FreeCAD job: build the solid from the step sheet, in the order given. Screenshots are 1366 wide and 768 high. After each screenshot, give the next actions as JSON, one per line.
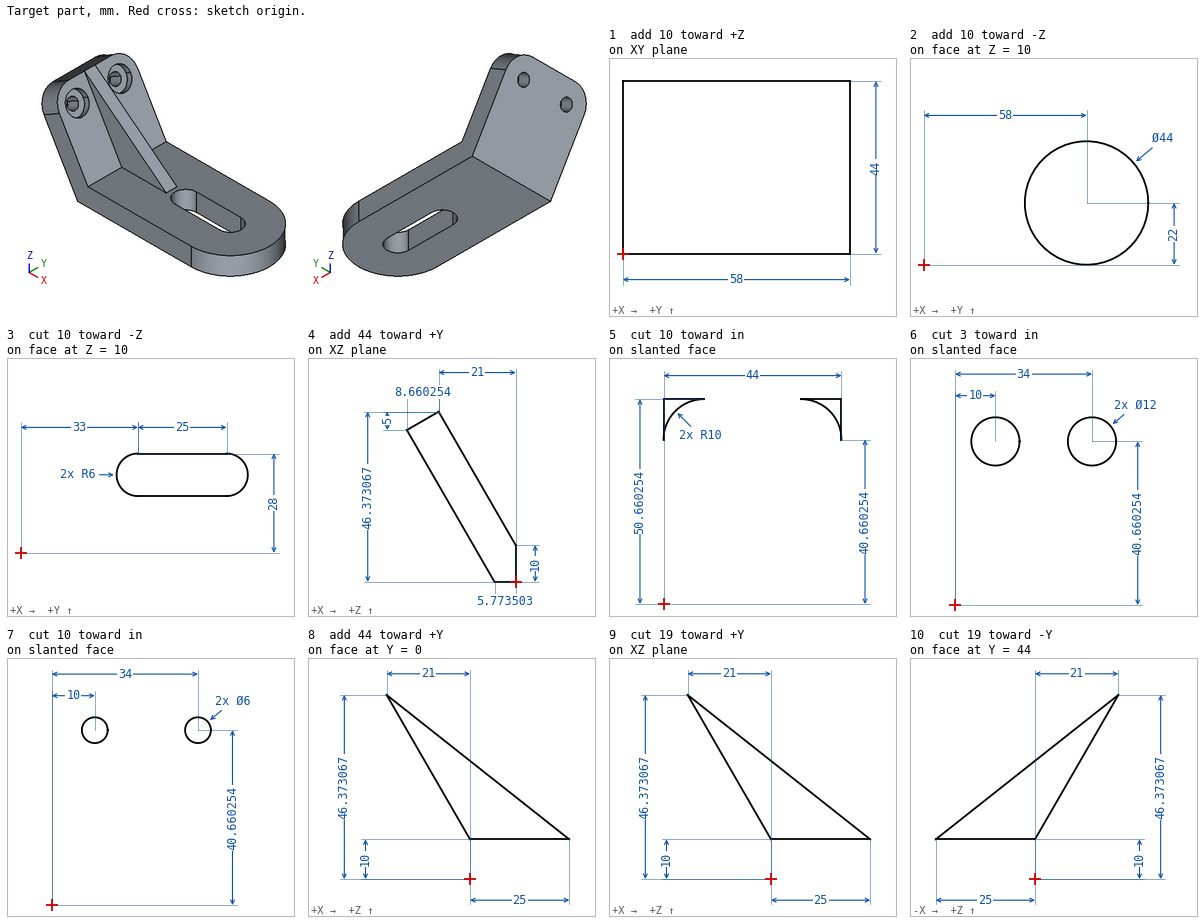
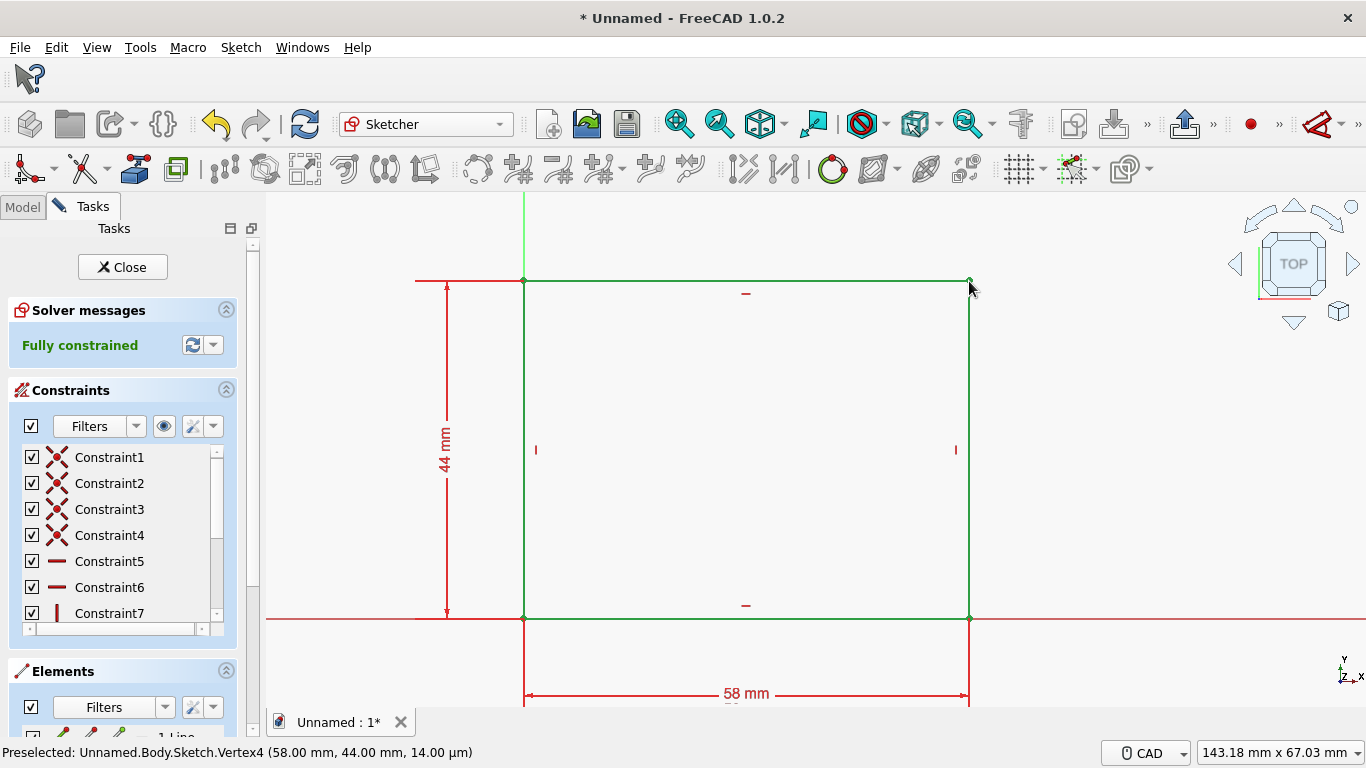
{"action": "left_click", "coordinate": [123, 267]}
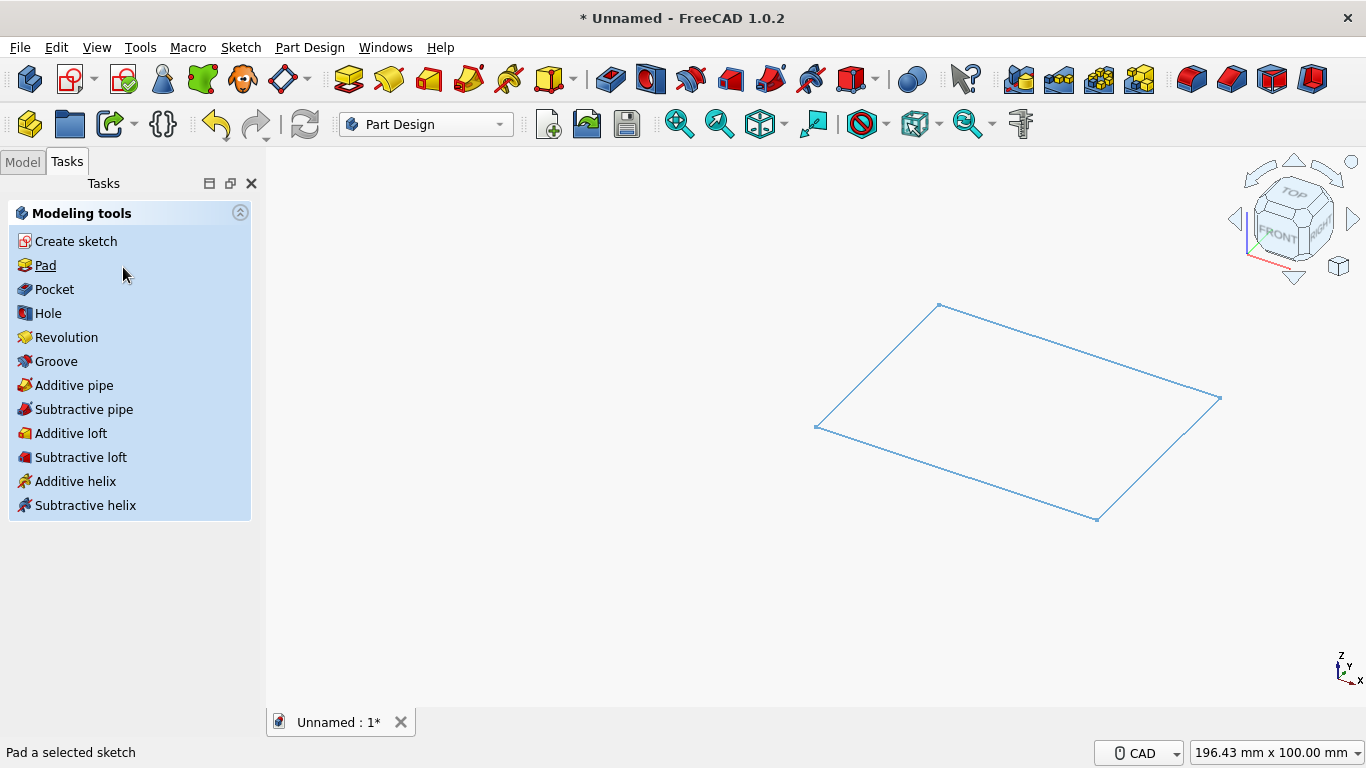
{"action": "left_click", "coordinate": [350, 80]}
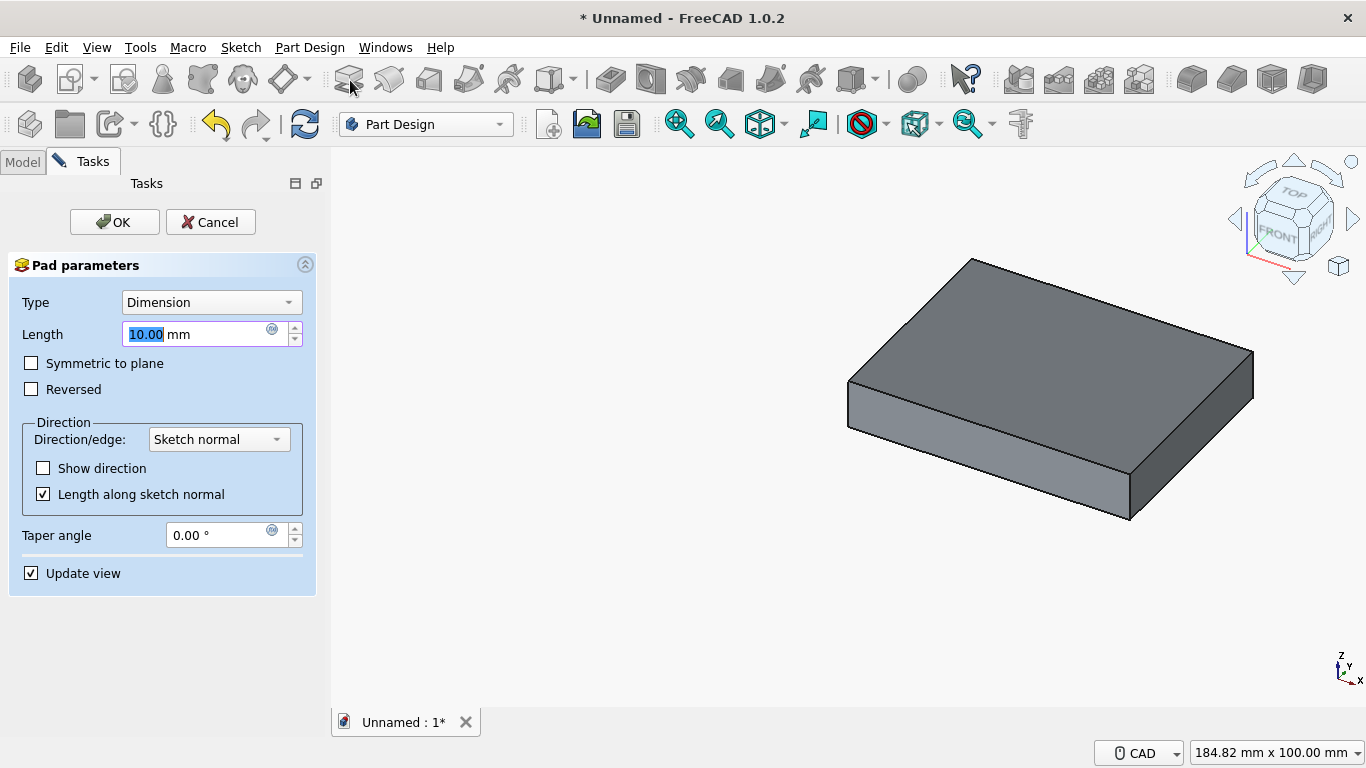
{"action": "type", "text": "10"}
{"action": "key", "text": "Tab"}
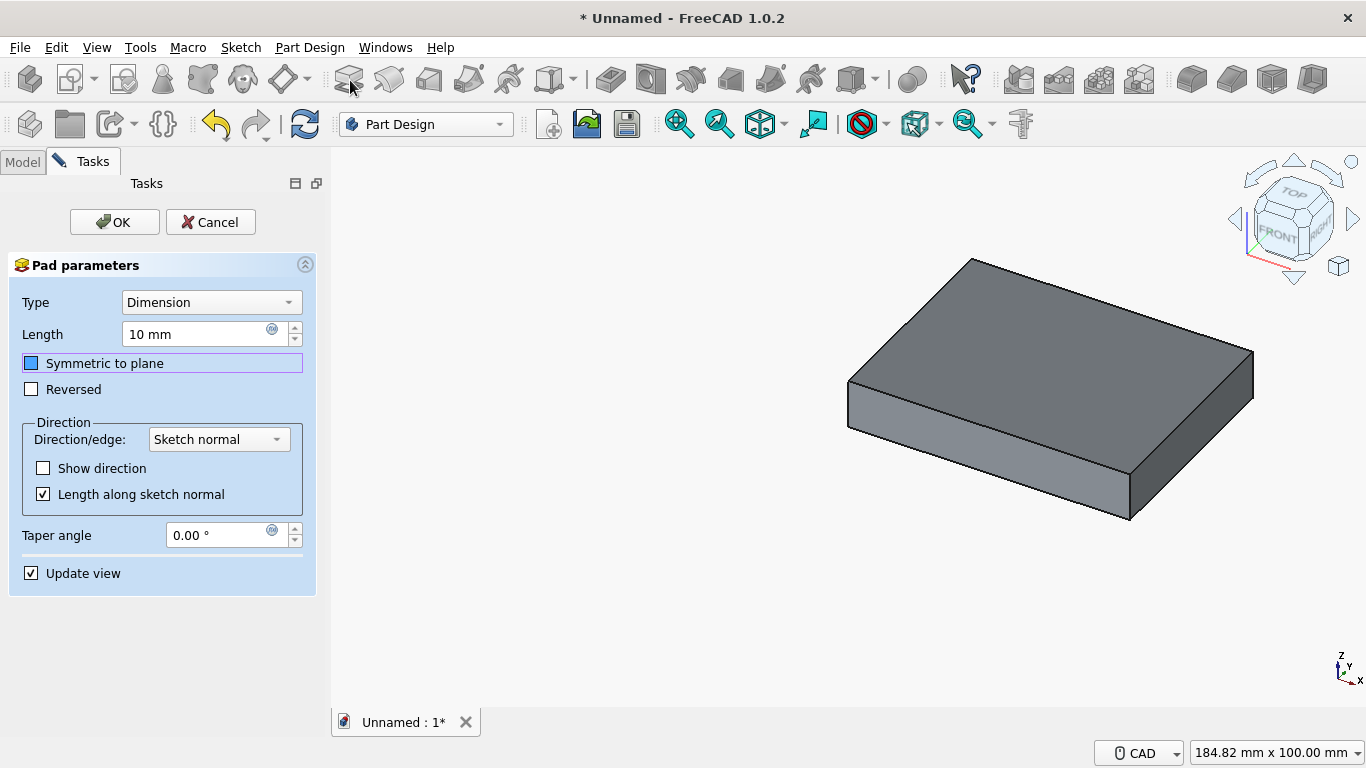
{"action": "left_click", "coordinate": [115, 222]}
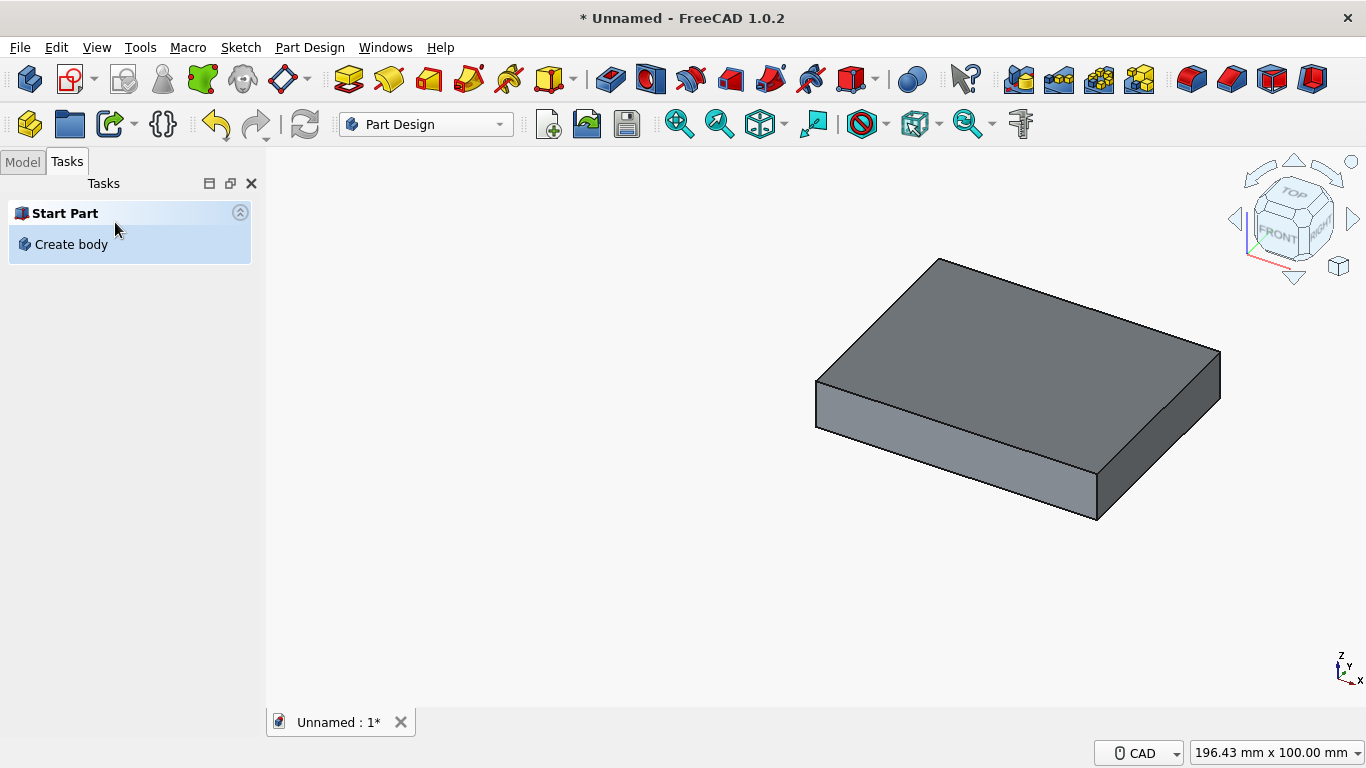
{"action": "left_click", "coordinate": [1018, 366]}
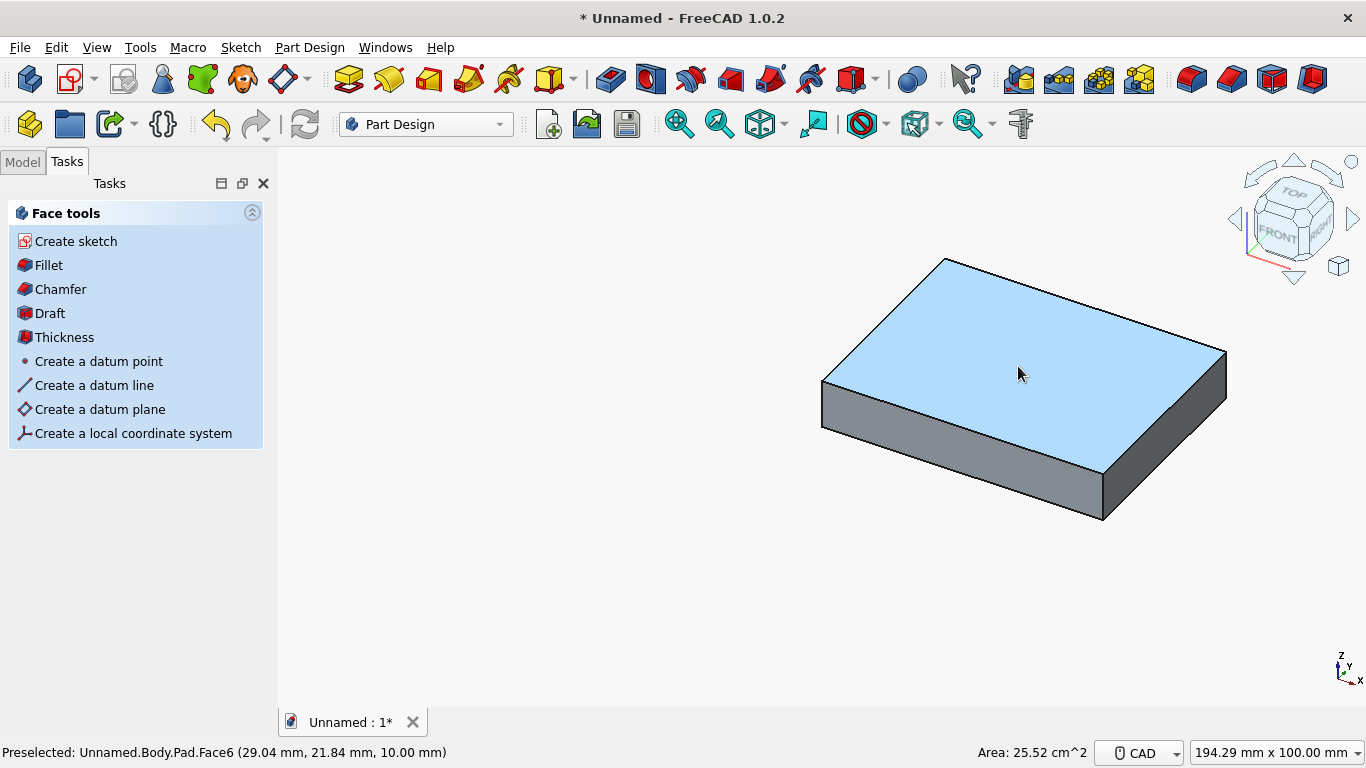
{"action": "left_click", "coordinate": [70, 80]}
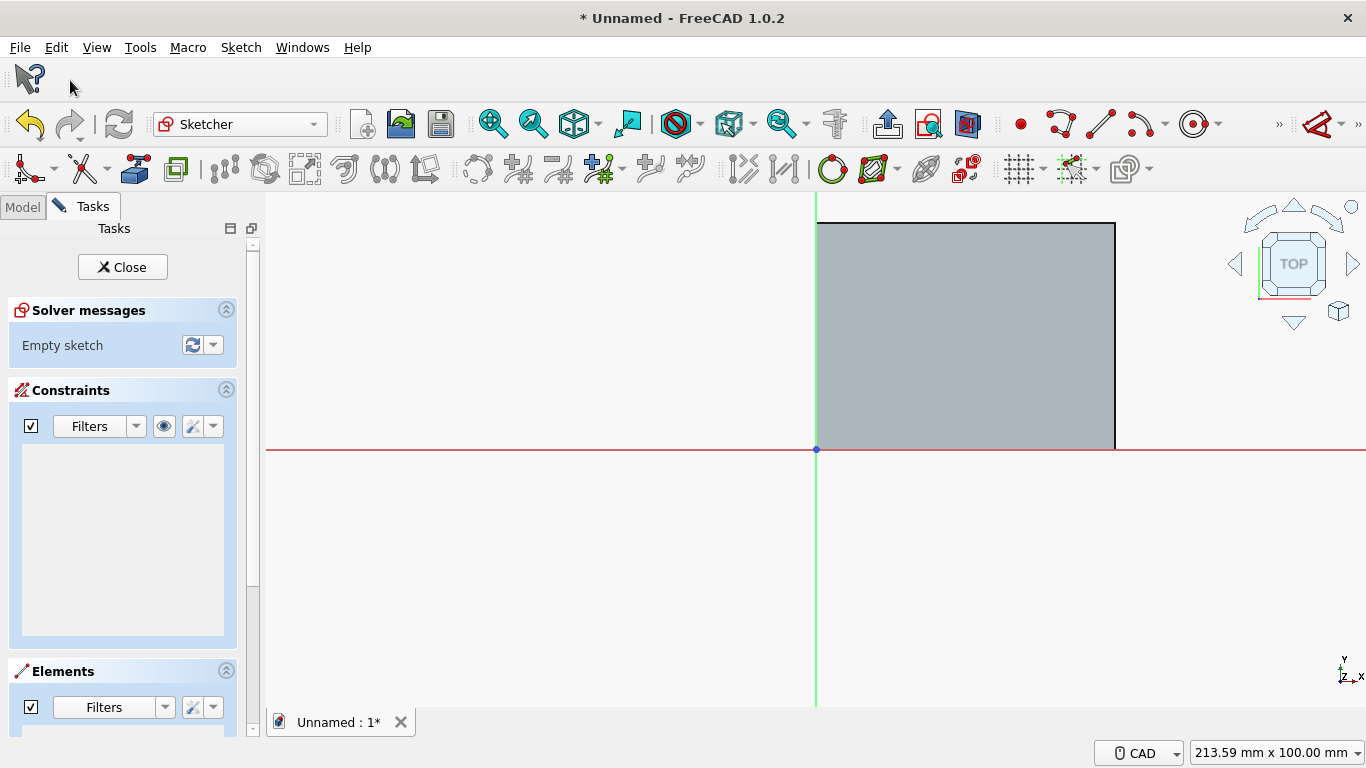
{"action": "scroll", "coordinate": [294, 679], "scroll_direction": "down", "scroll_amount": 1}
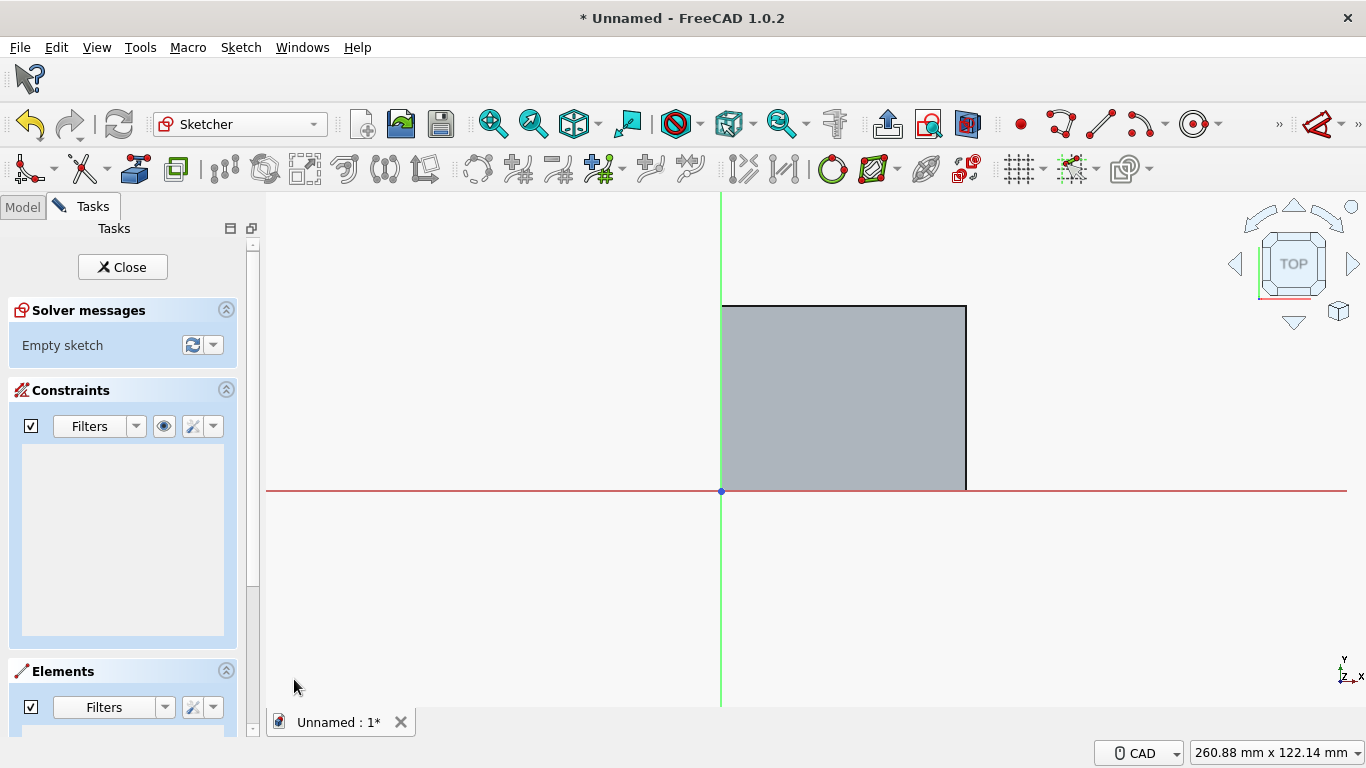
{"action": "scroll", "coordinate": [1063, 336], "scroll_direction": "up", "scroll_amount": 3}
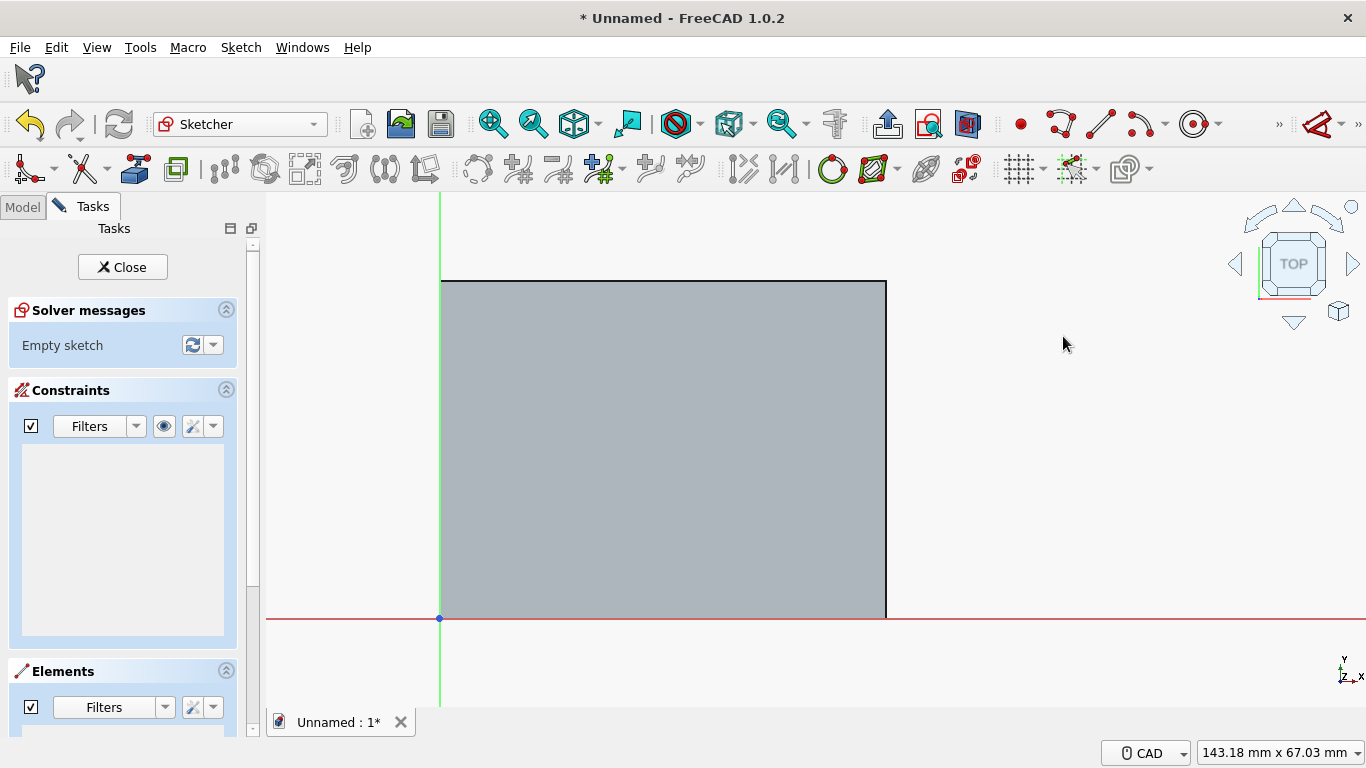
{"action": "left_click", "coordinate": [1194, 124]}